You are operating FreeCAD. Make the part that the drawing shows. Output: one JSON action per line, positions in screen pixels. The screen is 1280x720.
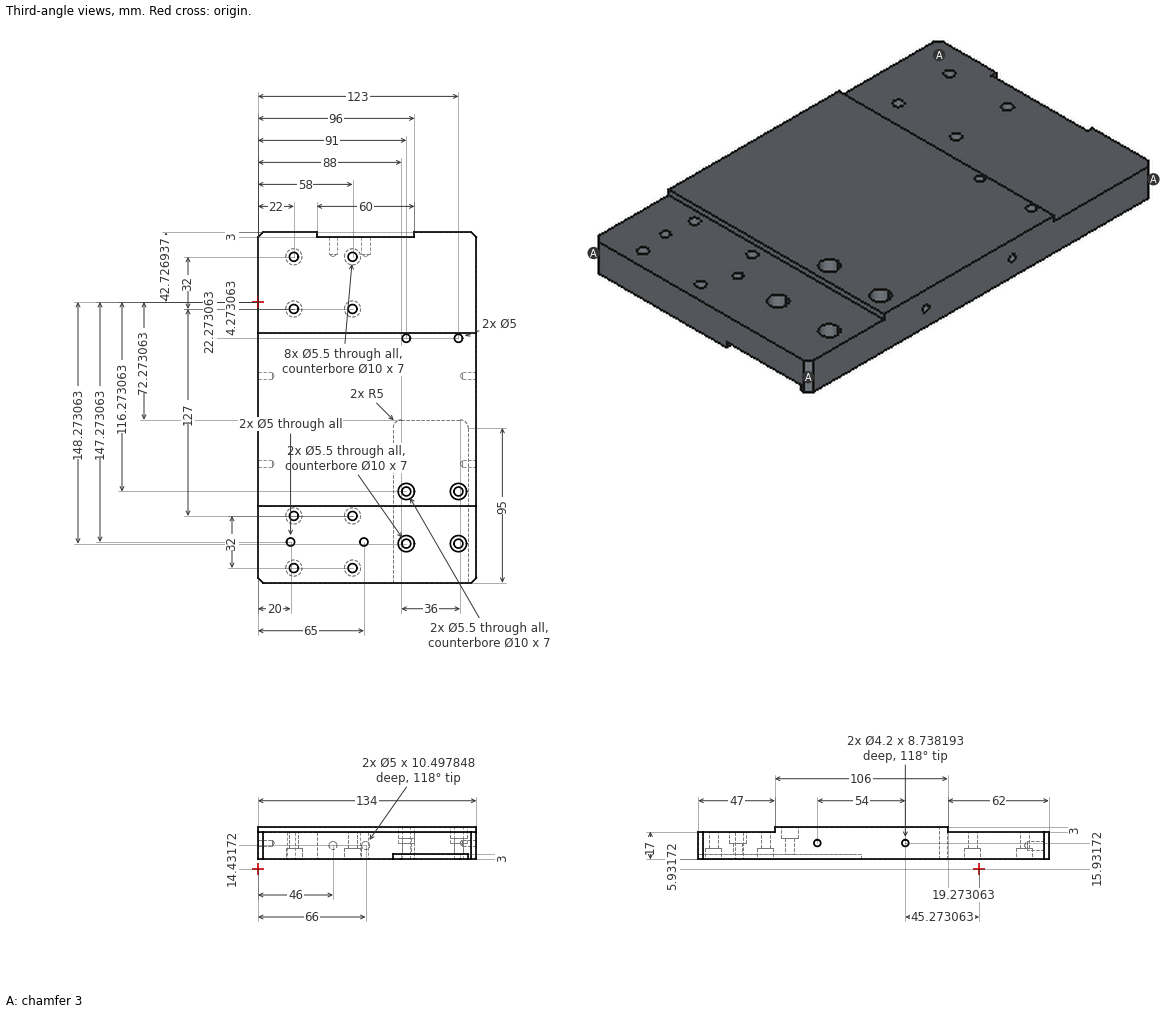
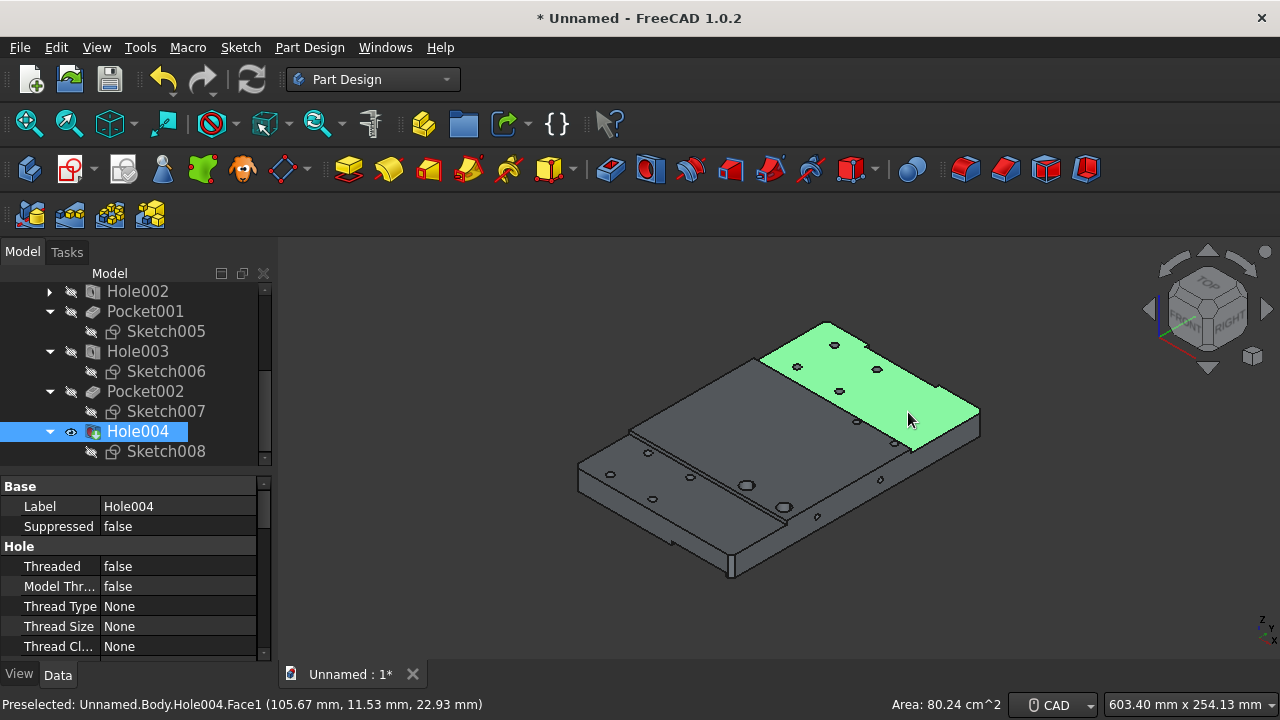
{"action": "left_click", "coordinate": [70, 170]}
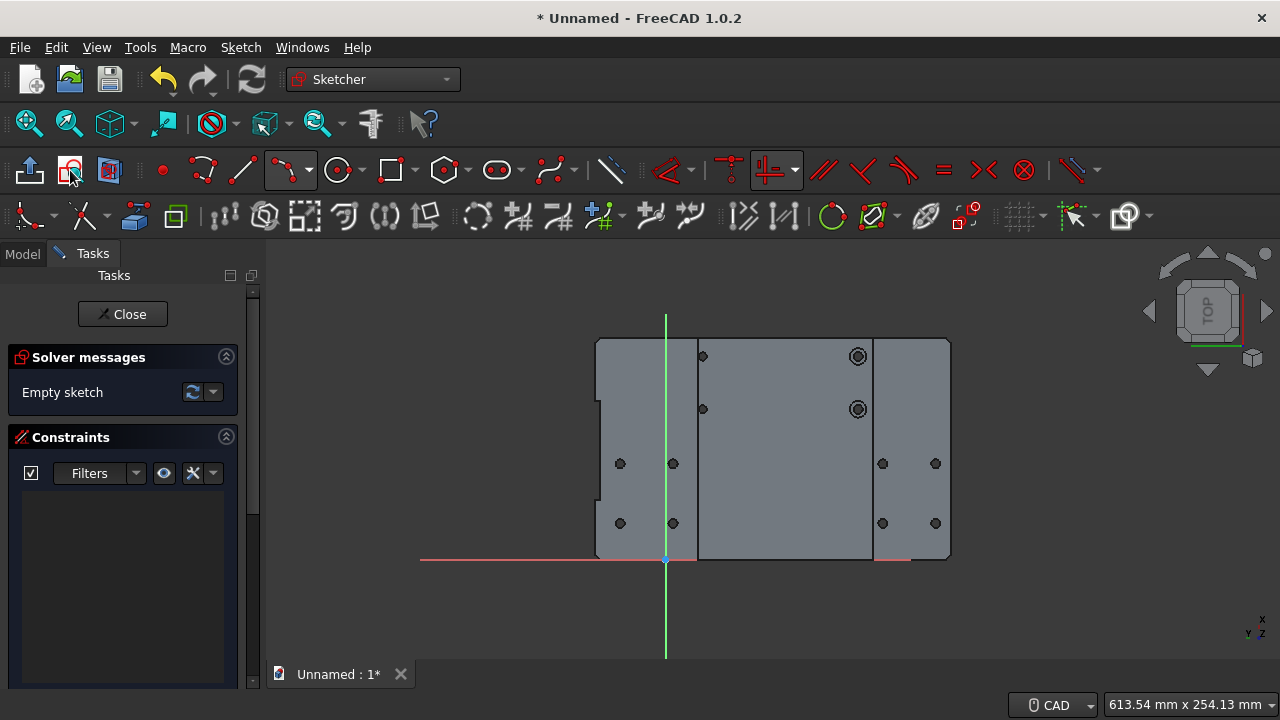
{"action": "scroll", "coordinate": [979, 361], "scroll_direction": "up", "scroll_amount": 7}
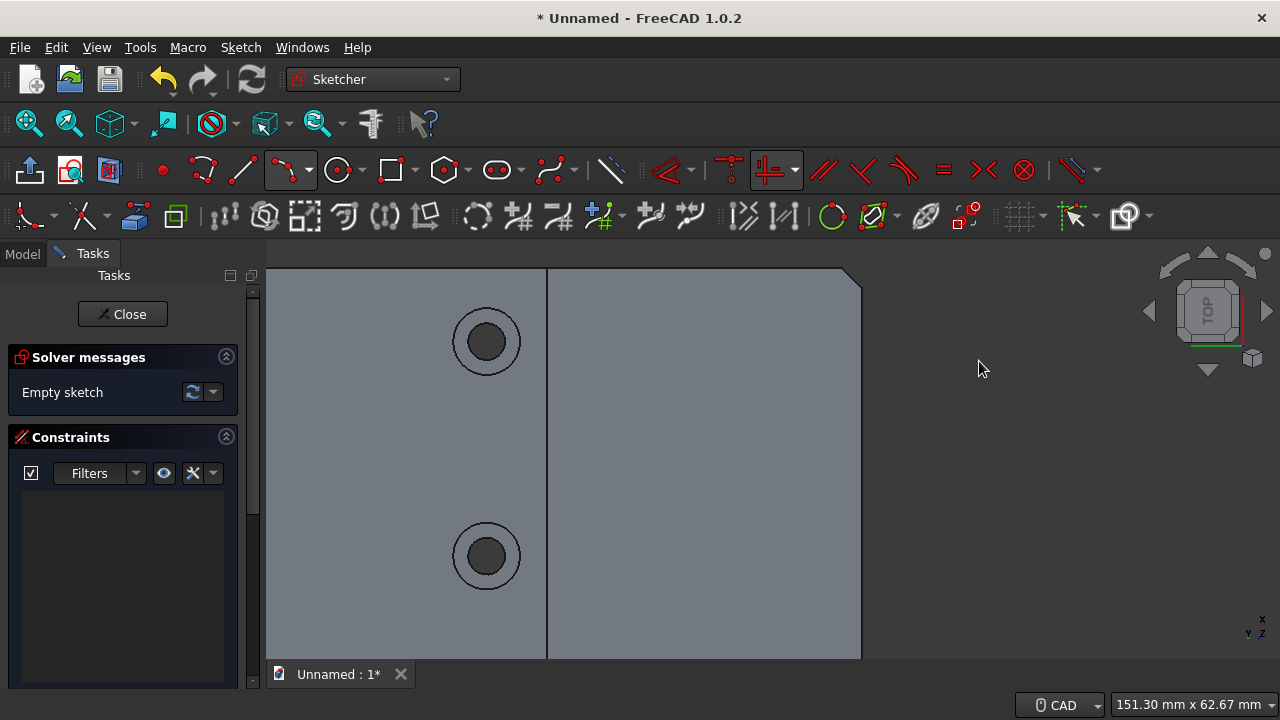
{"action": "left_click", "coordinate": [338, 170]}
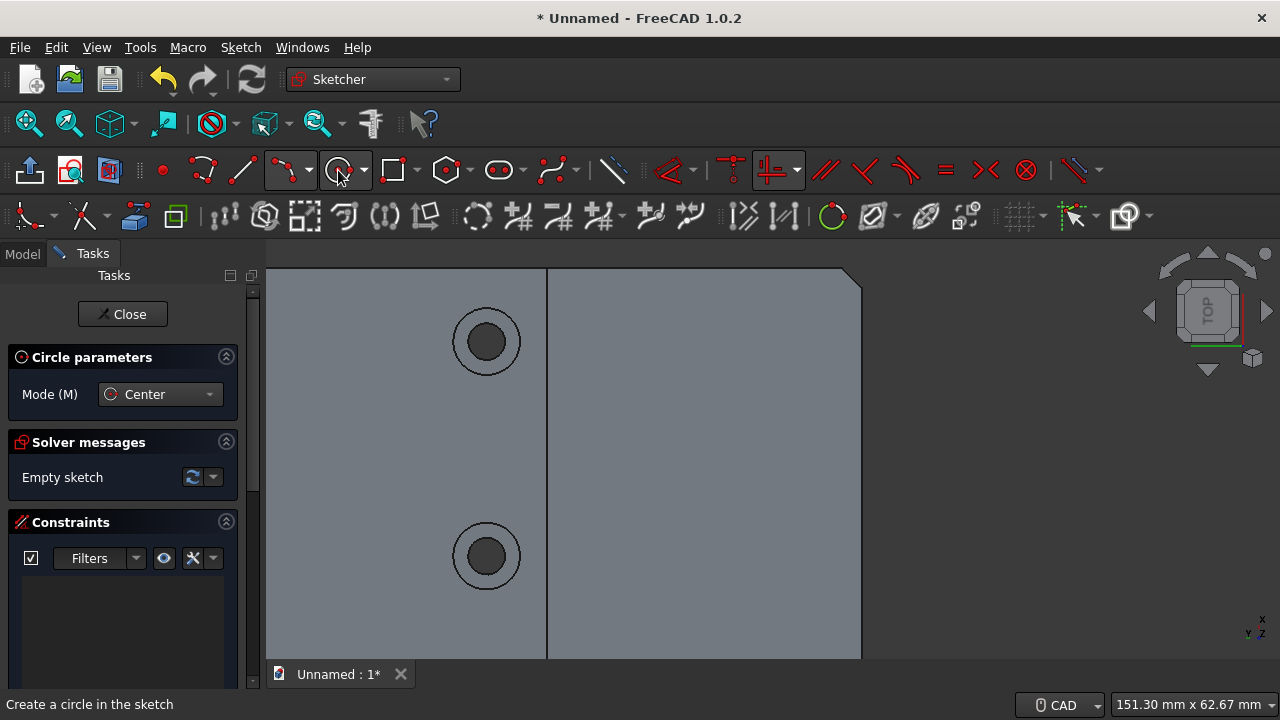
{"action": "scroll", "coordinate": [701, 556], "scroll_direction": "up", "scroll_amount": 2}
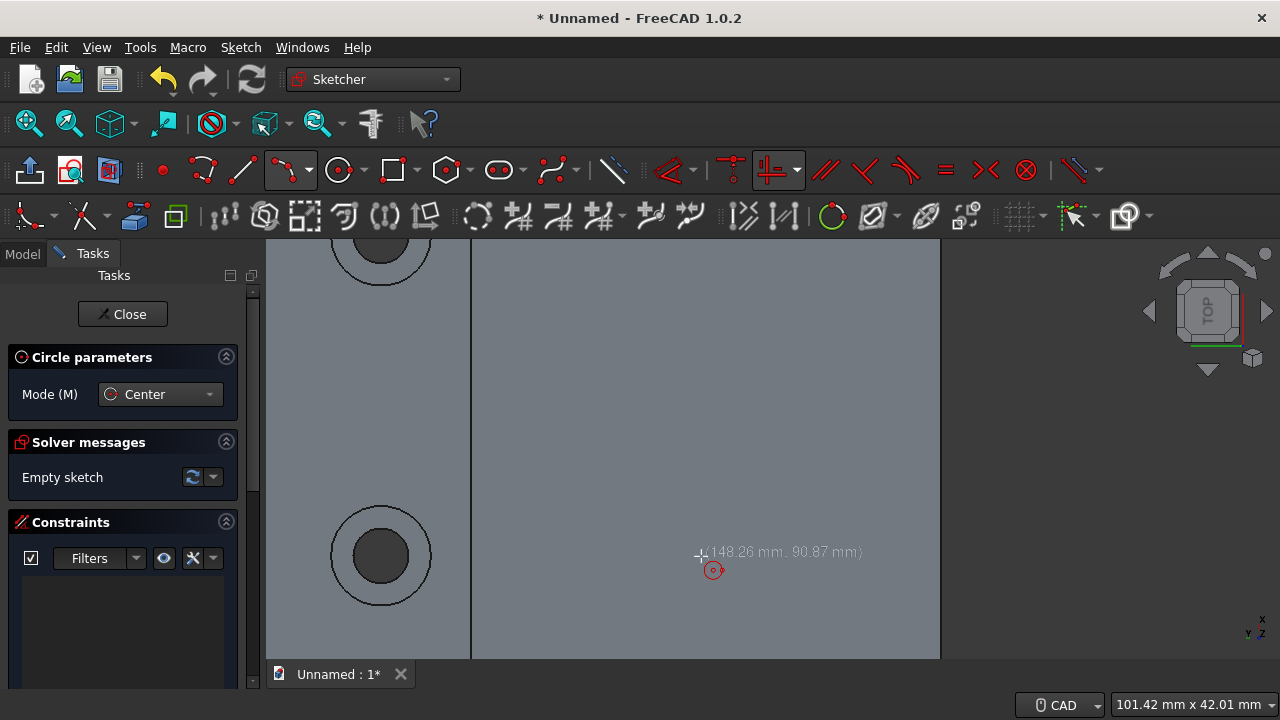
{"action": "left_click", "coordinate": [701, 556]}
{"action": "mouse_move", "coordinate": [720, 536]}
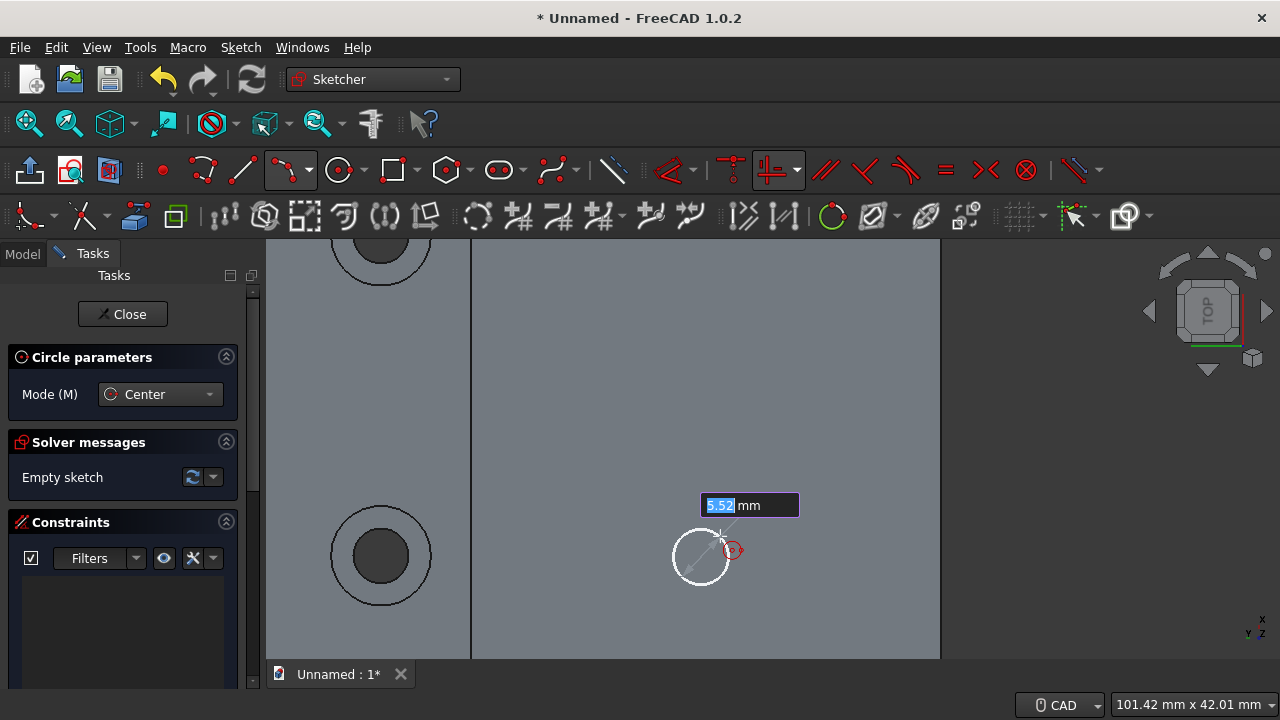
{"action": "type", "text": "5.5"}
{"action": "key", "text": "Return"}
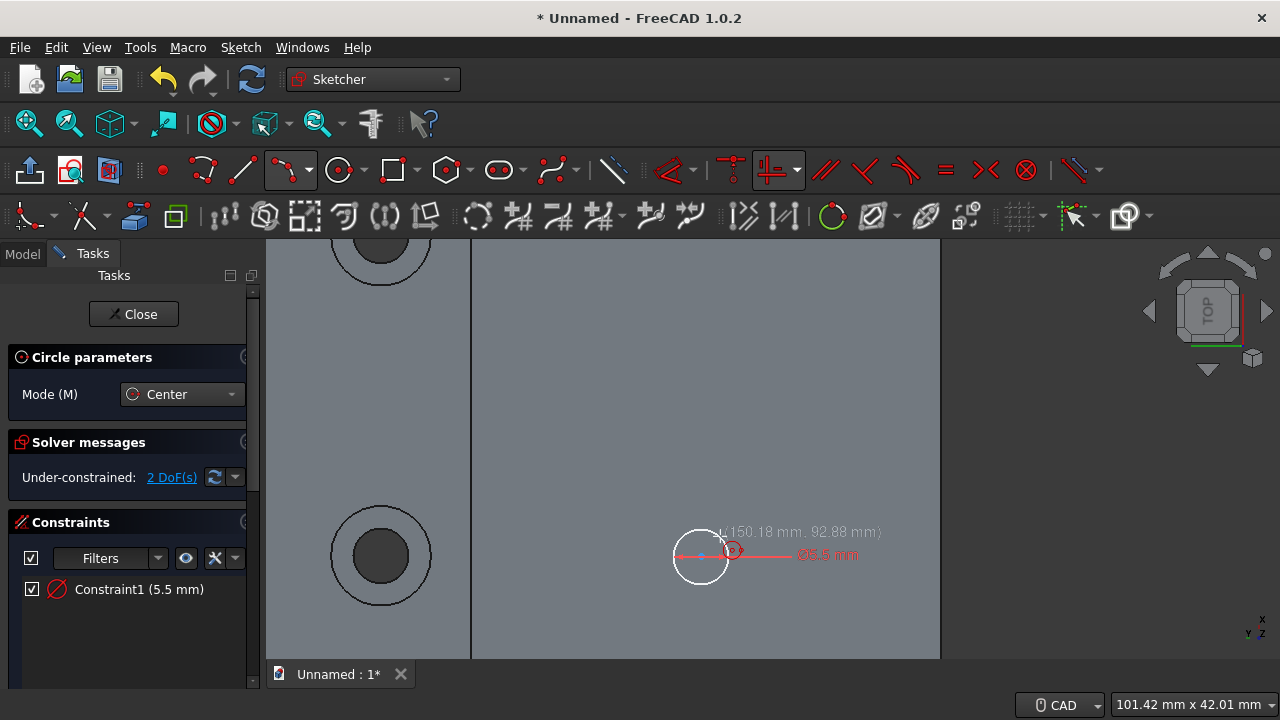
{"action": "scroll", "coordinate": [712, 557], "scroll_direction": "down", "scroll_amount": 2}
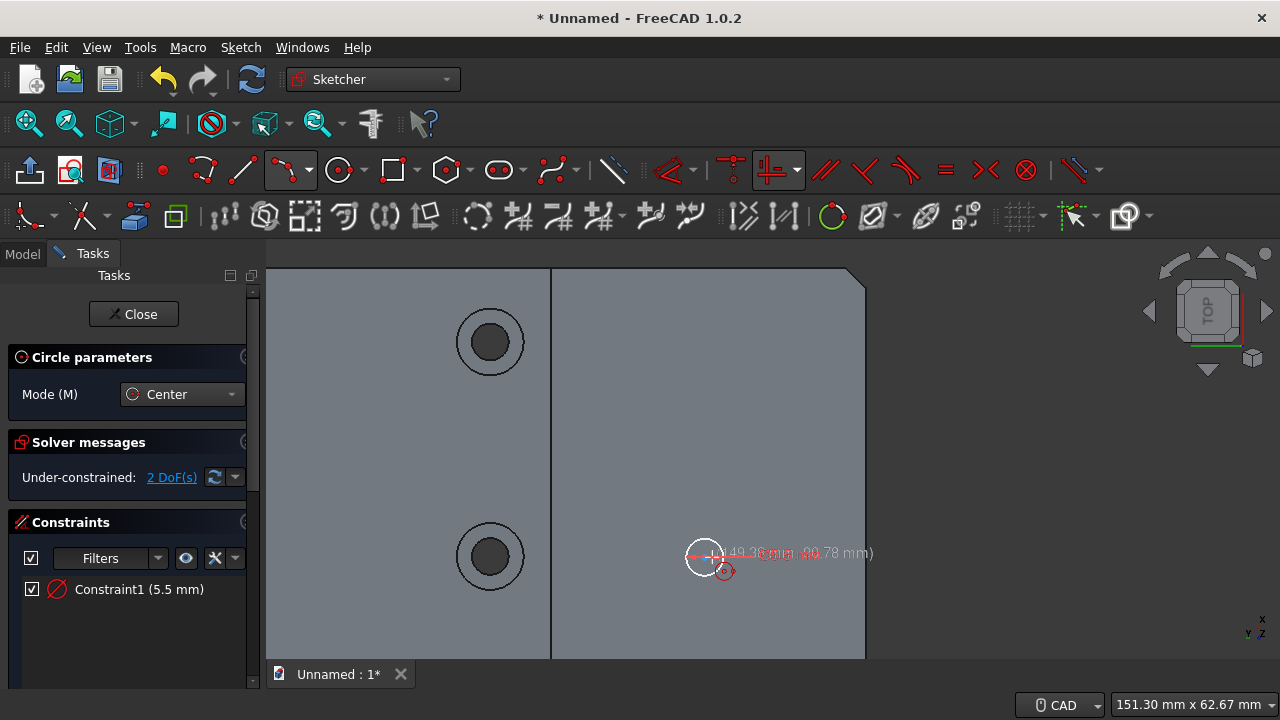
{"action": "scroll", "coordinate": [705, 342], "scroll_direction": "up", "scroll_amount": 2}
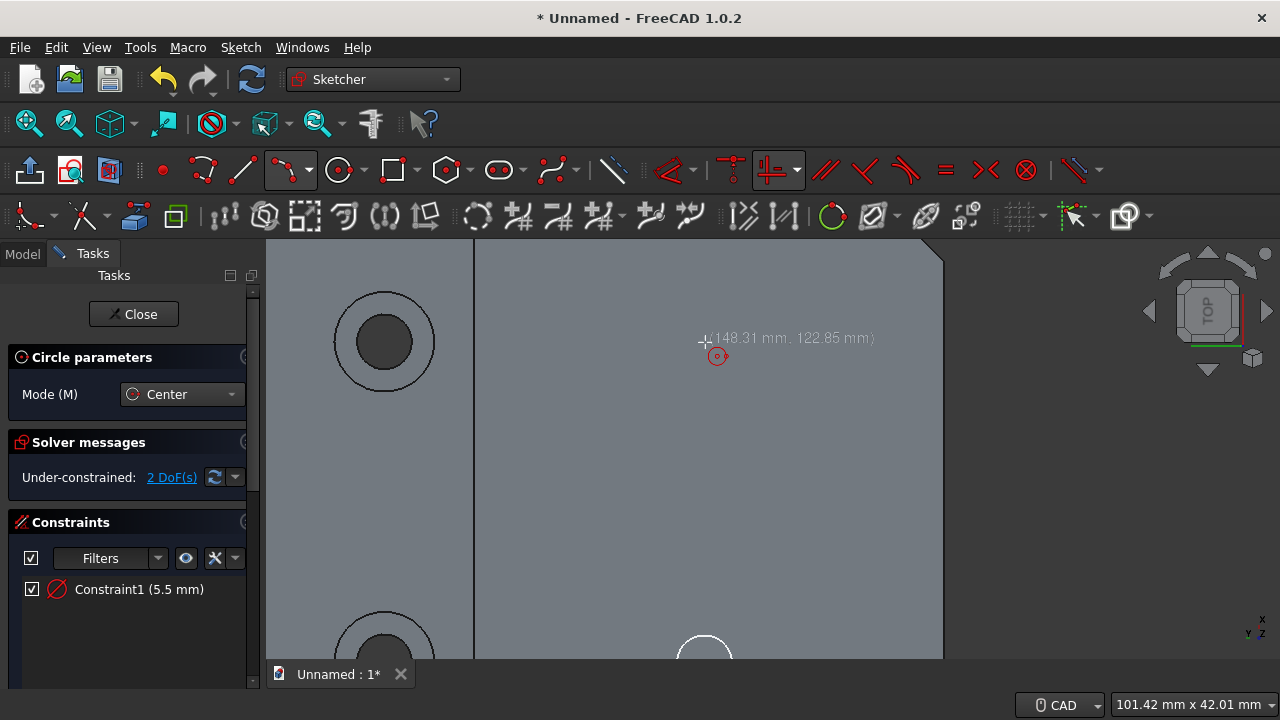
{"action": "left_click", "coordinate": [704, 342]}
{"action": "mouse_move", "coordinate": [724, 322]}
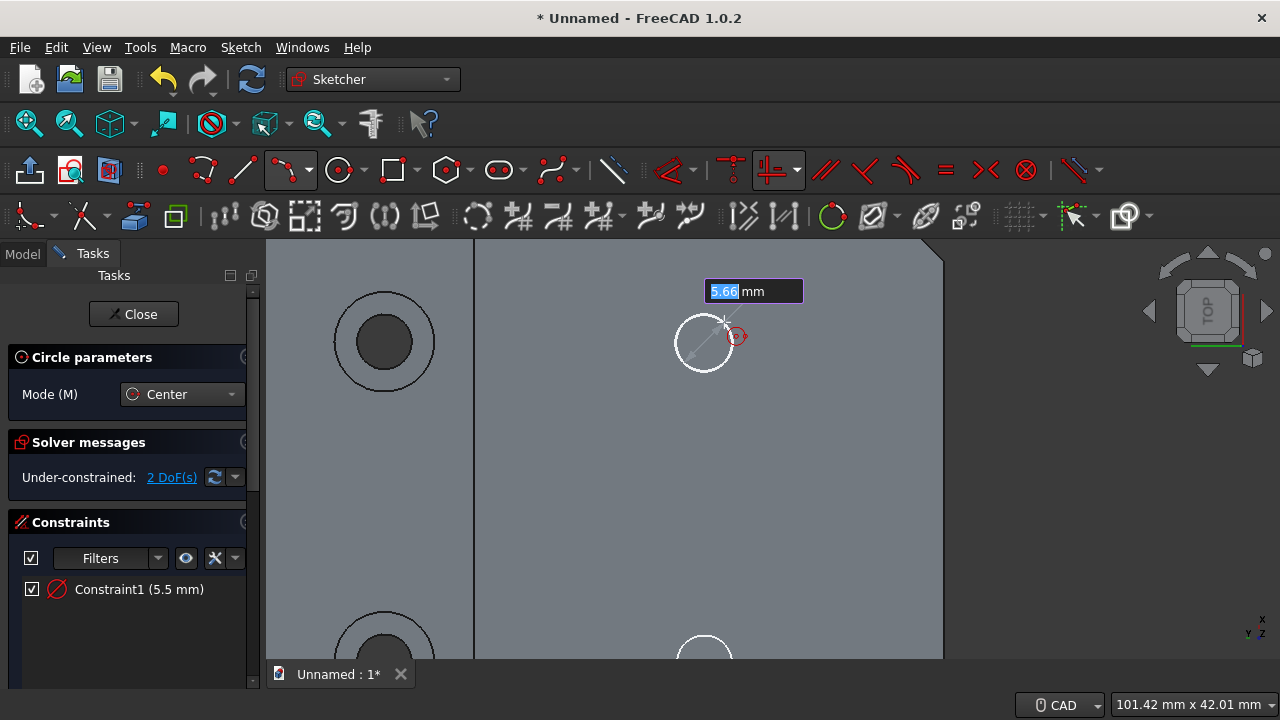
{"action": "type", "text": "5.5"}
{"action": "key", "text": "Return"}
{"action": "key", "text": "Escape"}